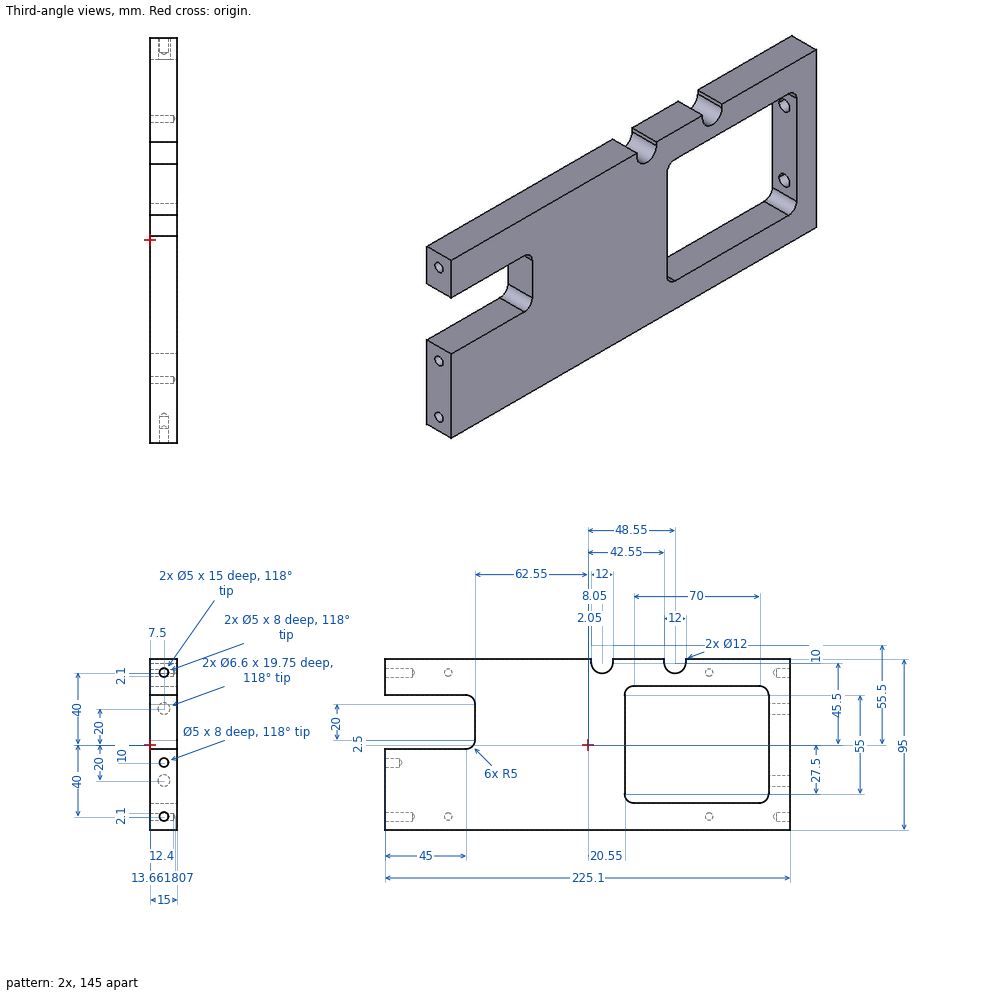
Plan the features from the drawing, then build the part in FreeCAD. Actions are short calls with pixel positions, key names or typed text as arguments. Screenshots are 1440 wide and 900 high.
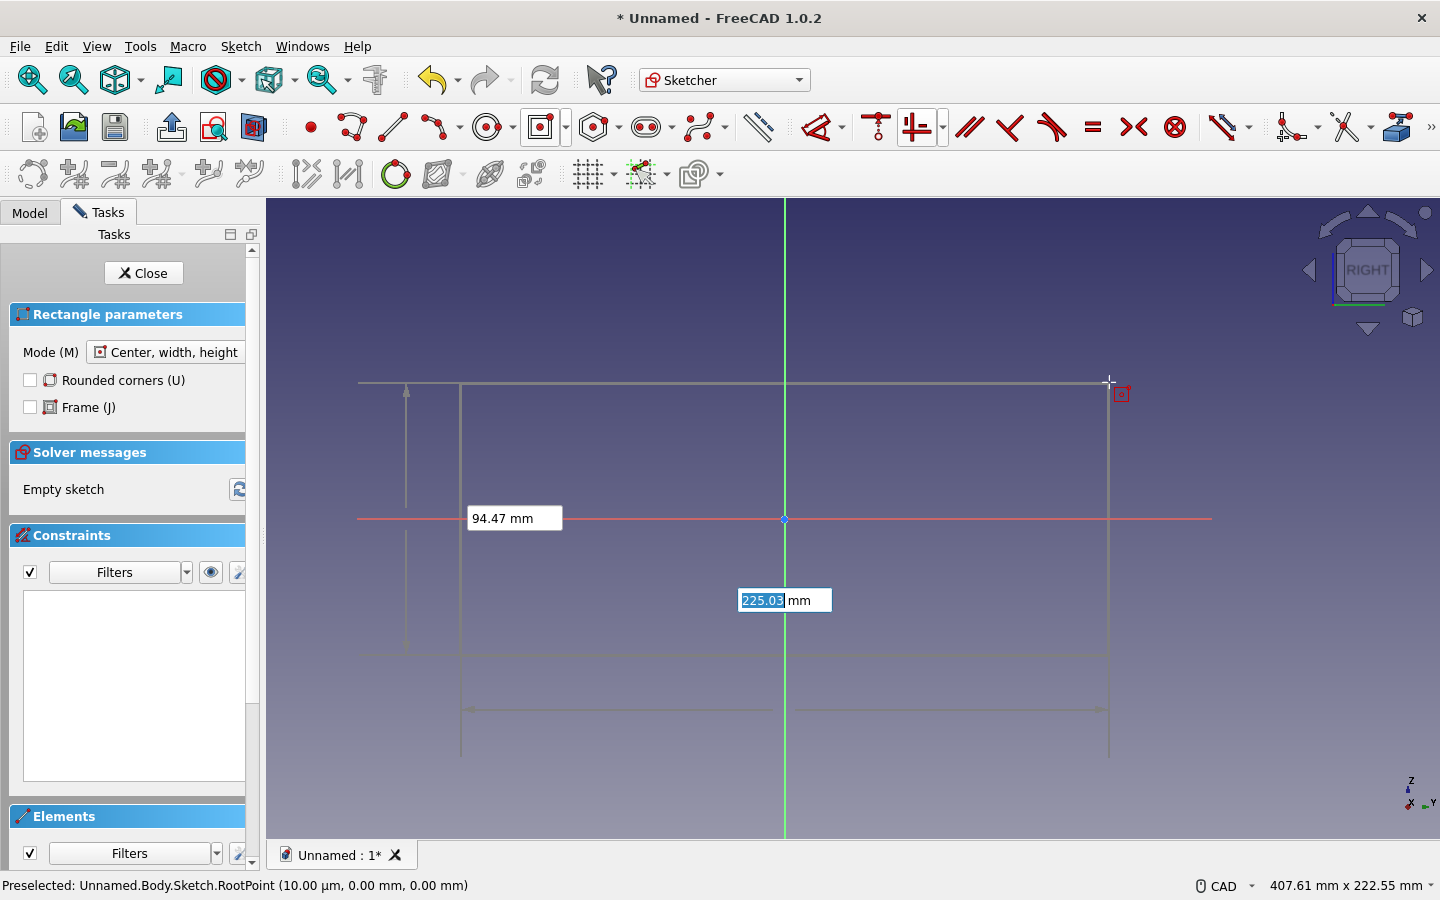
text(225.1)
key(Tab)
text(95)
key(Return)
key(Escape)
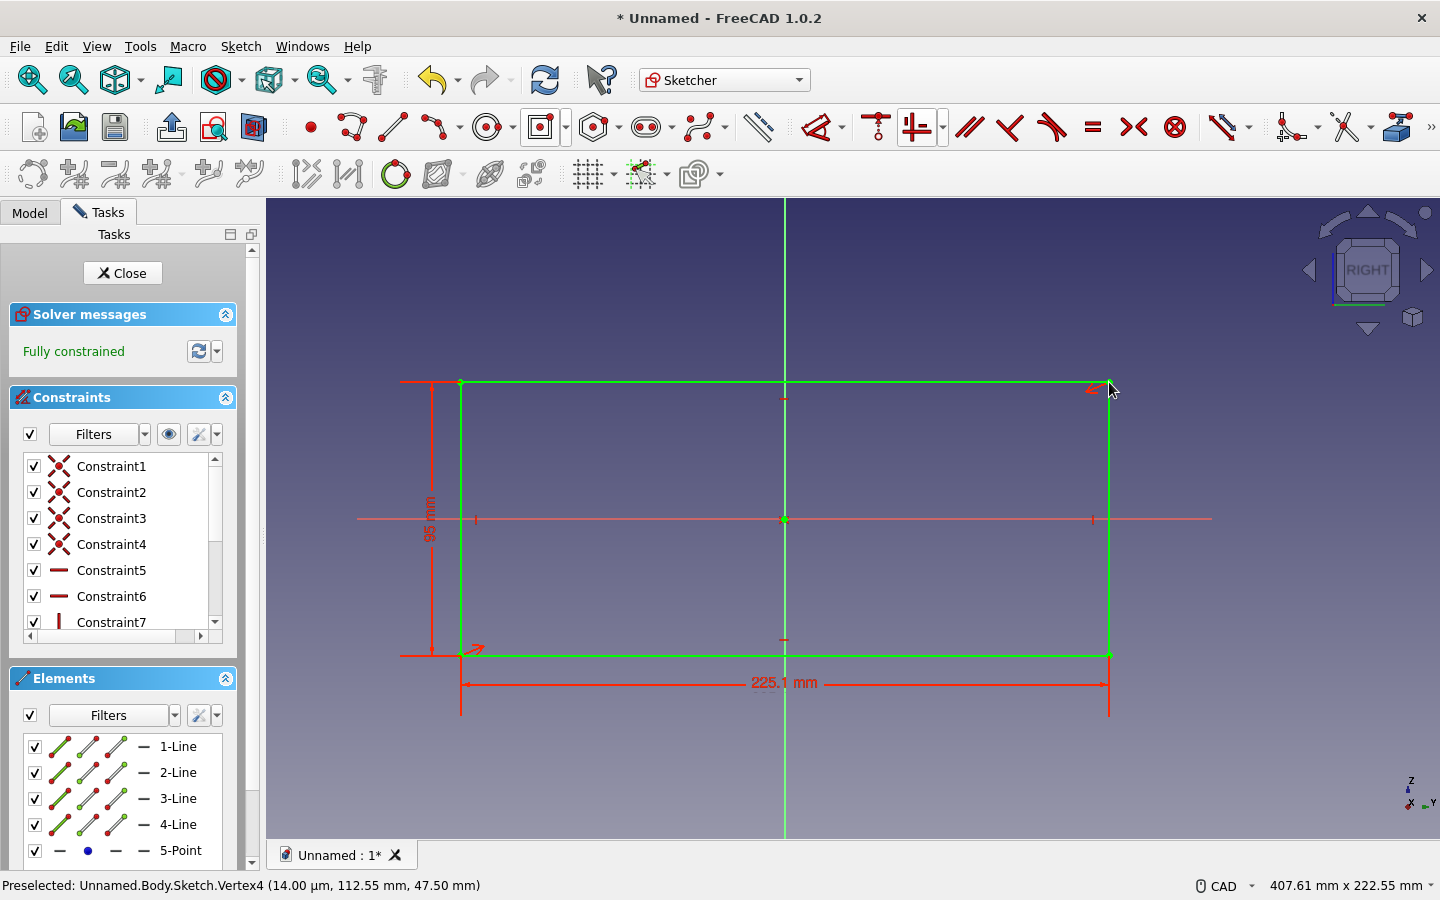
click(123, 273)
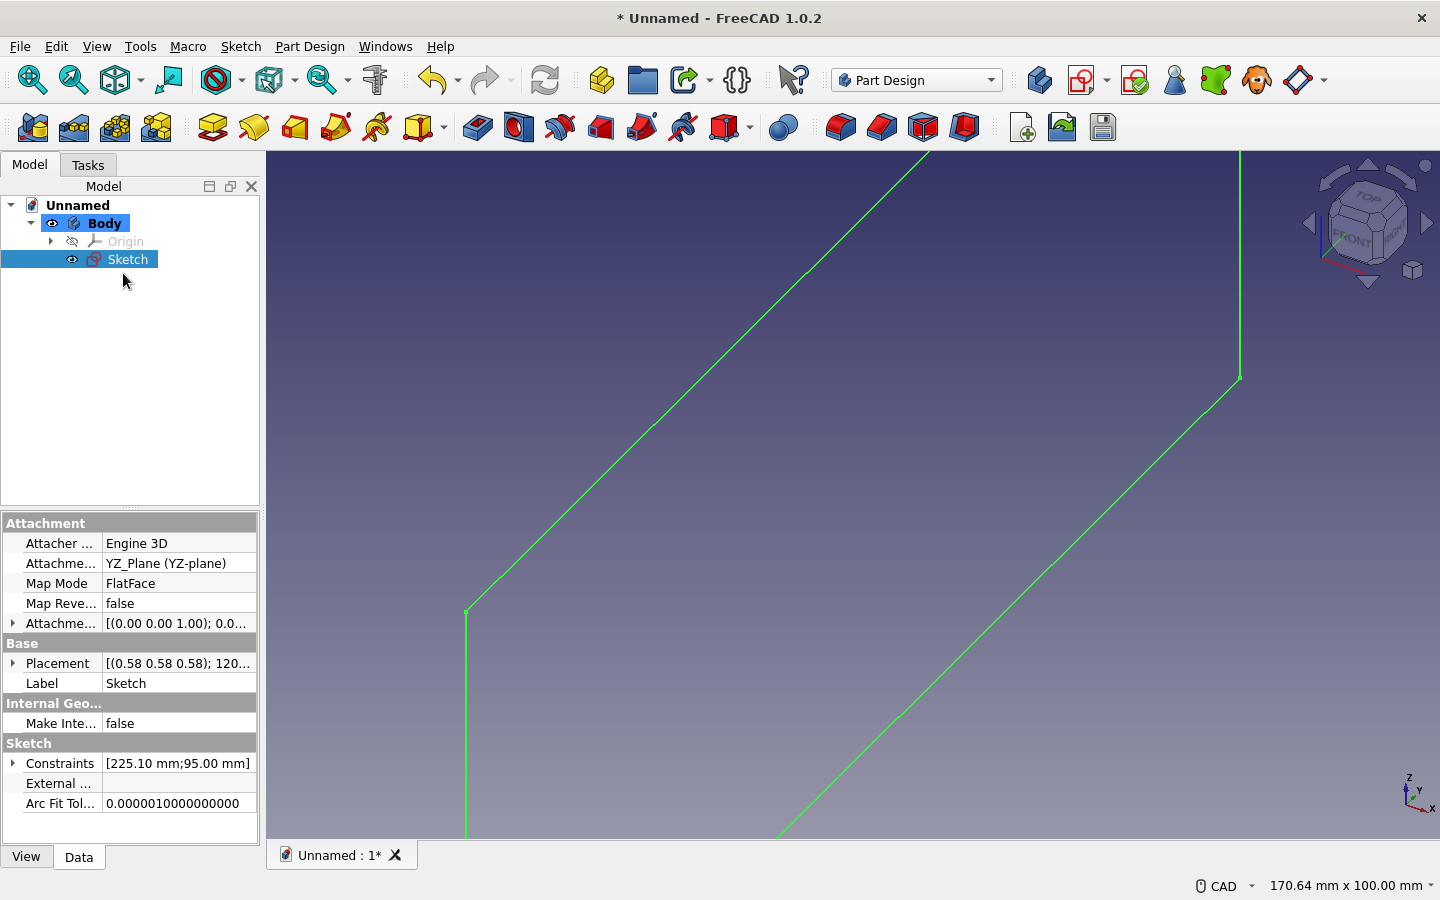
click(213, 128)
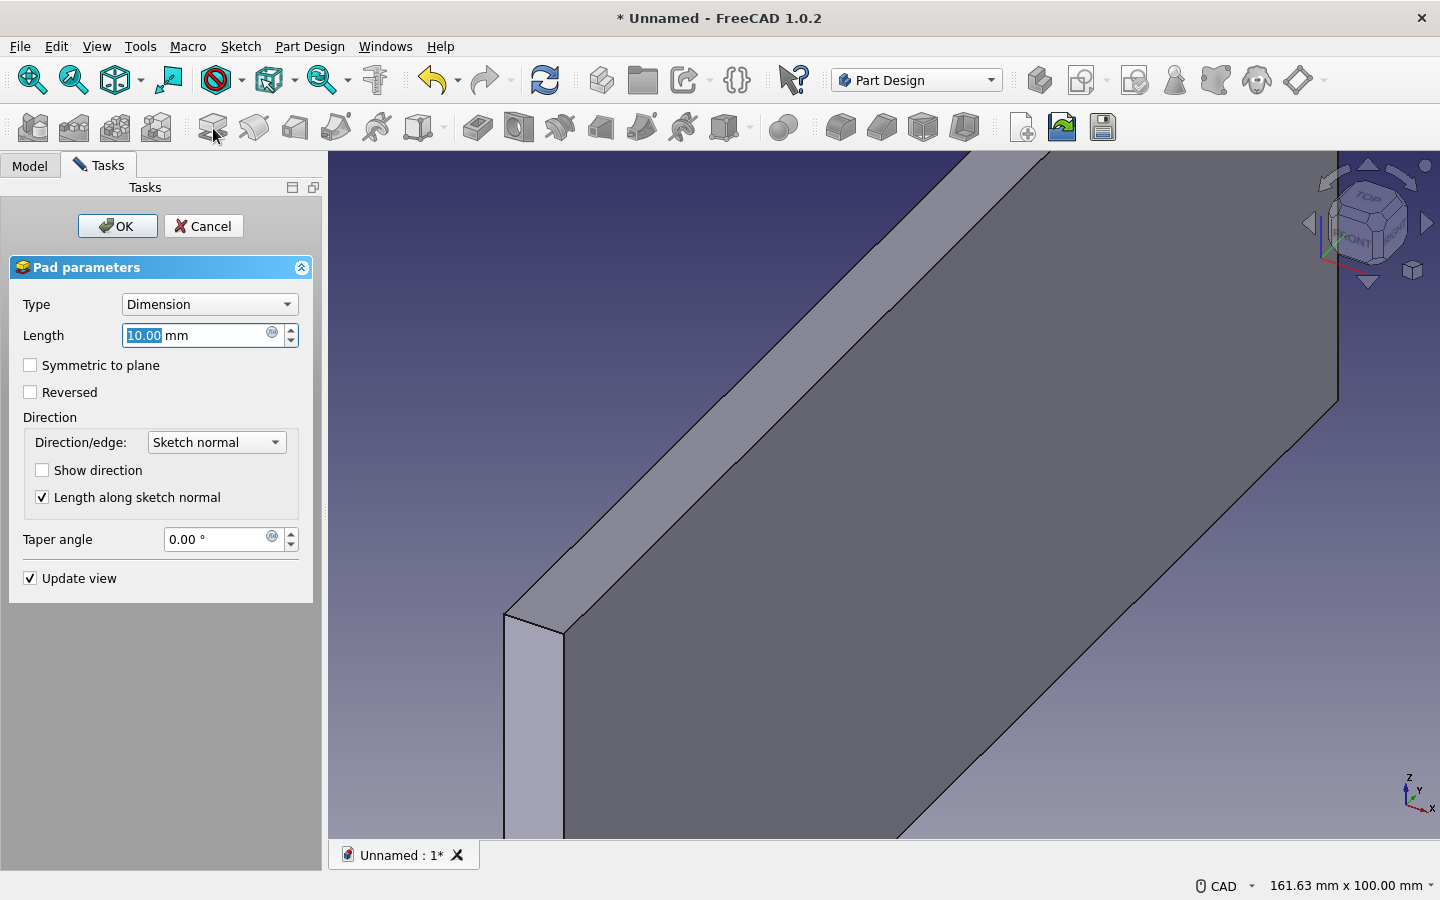
text(15)
key(Tab)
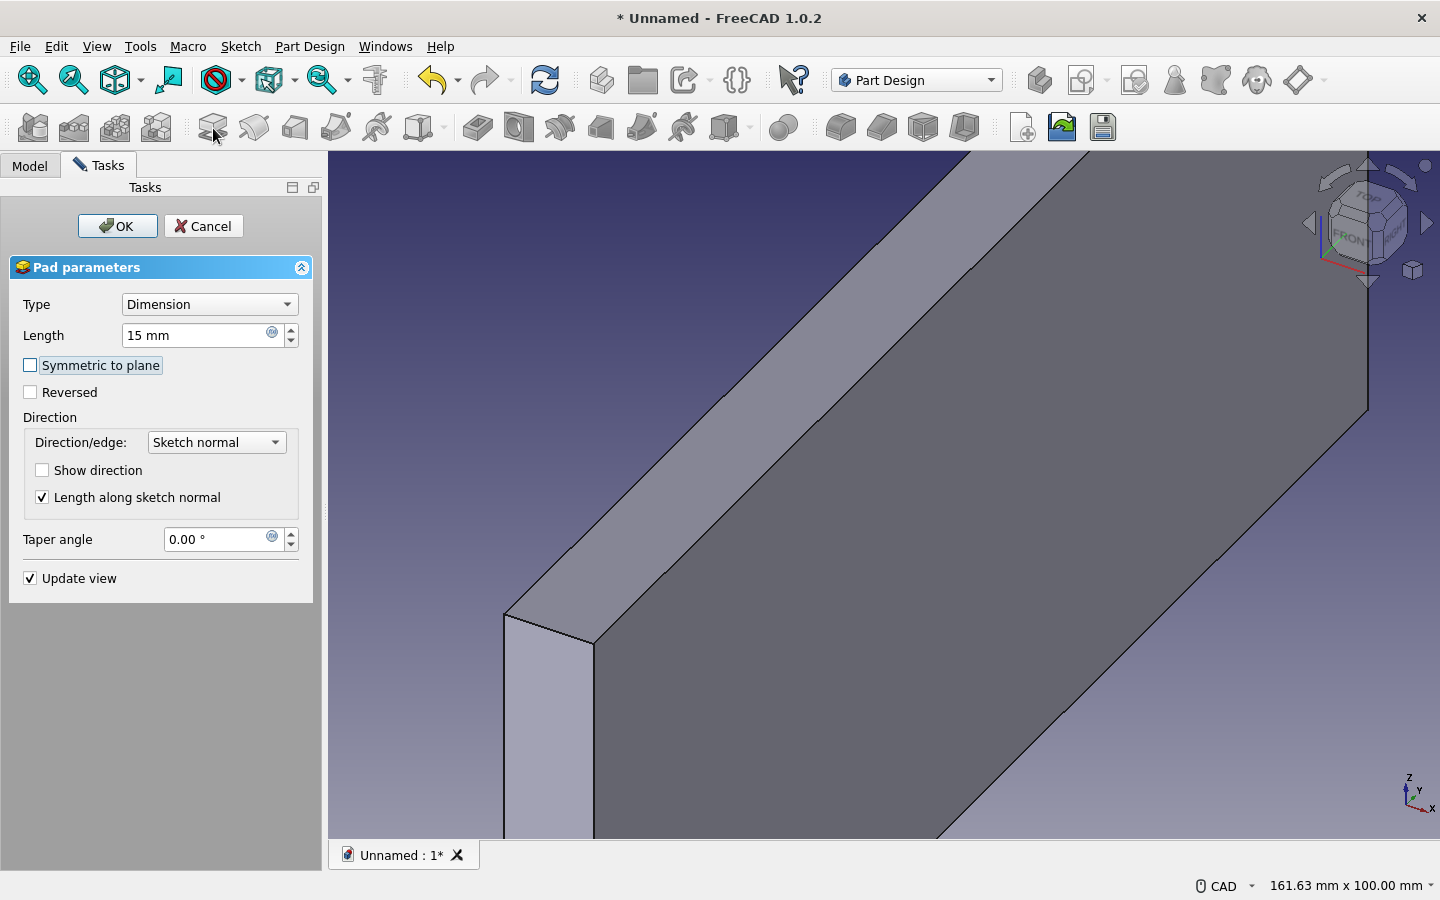
click(118, 226)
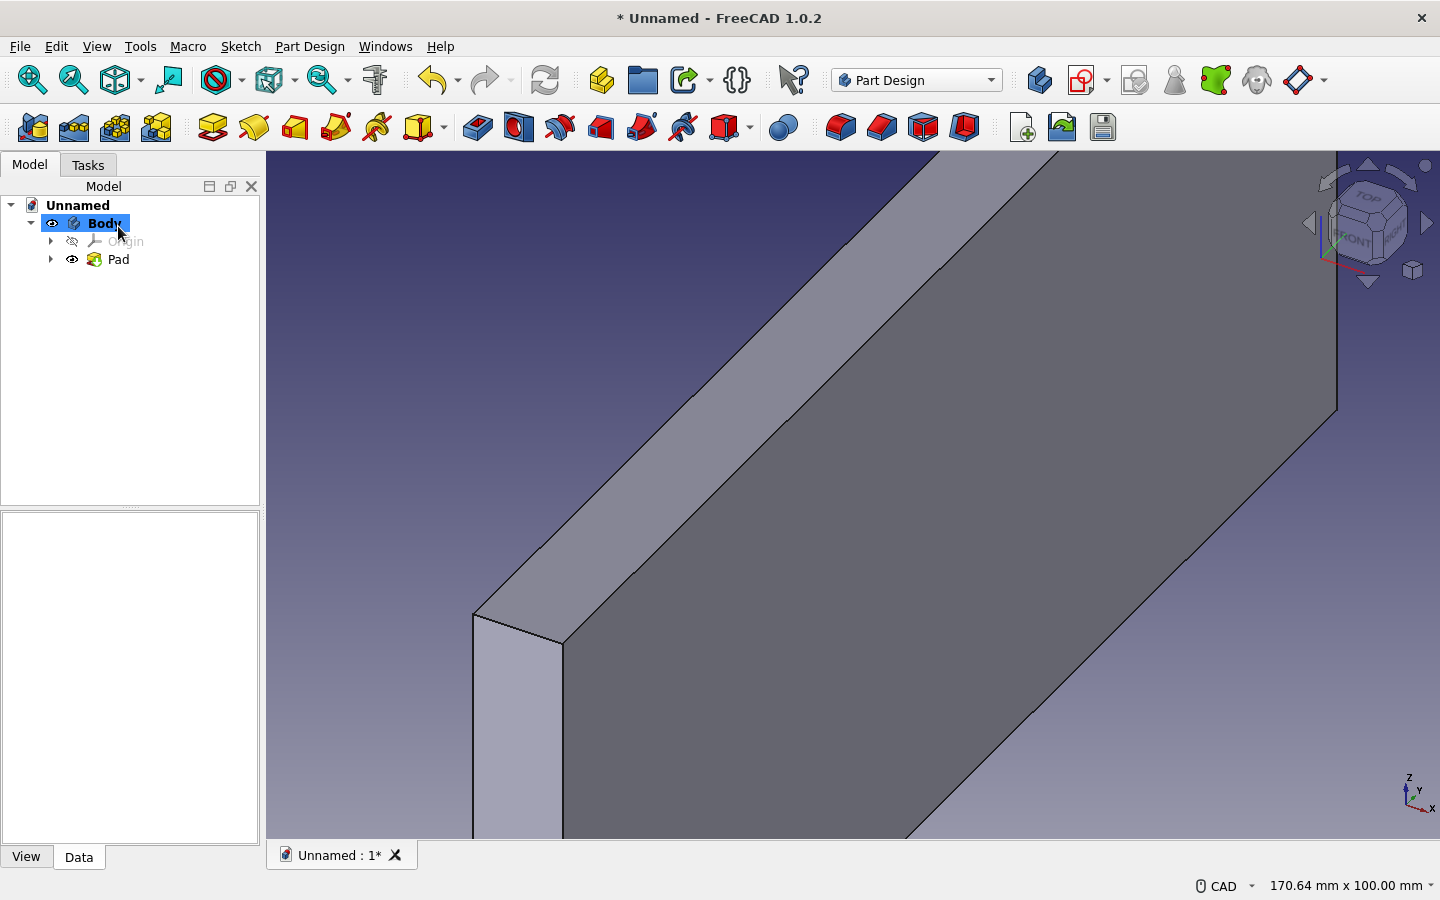
click(33, 80)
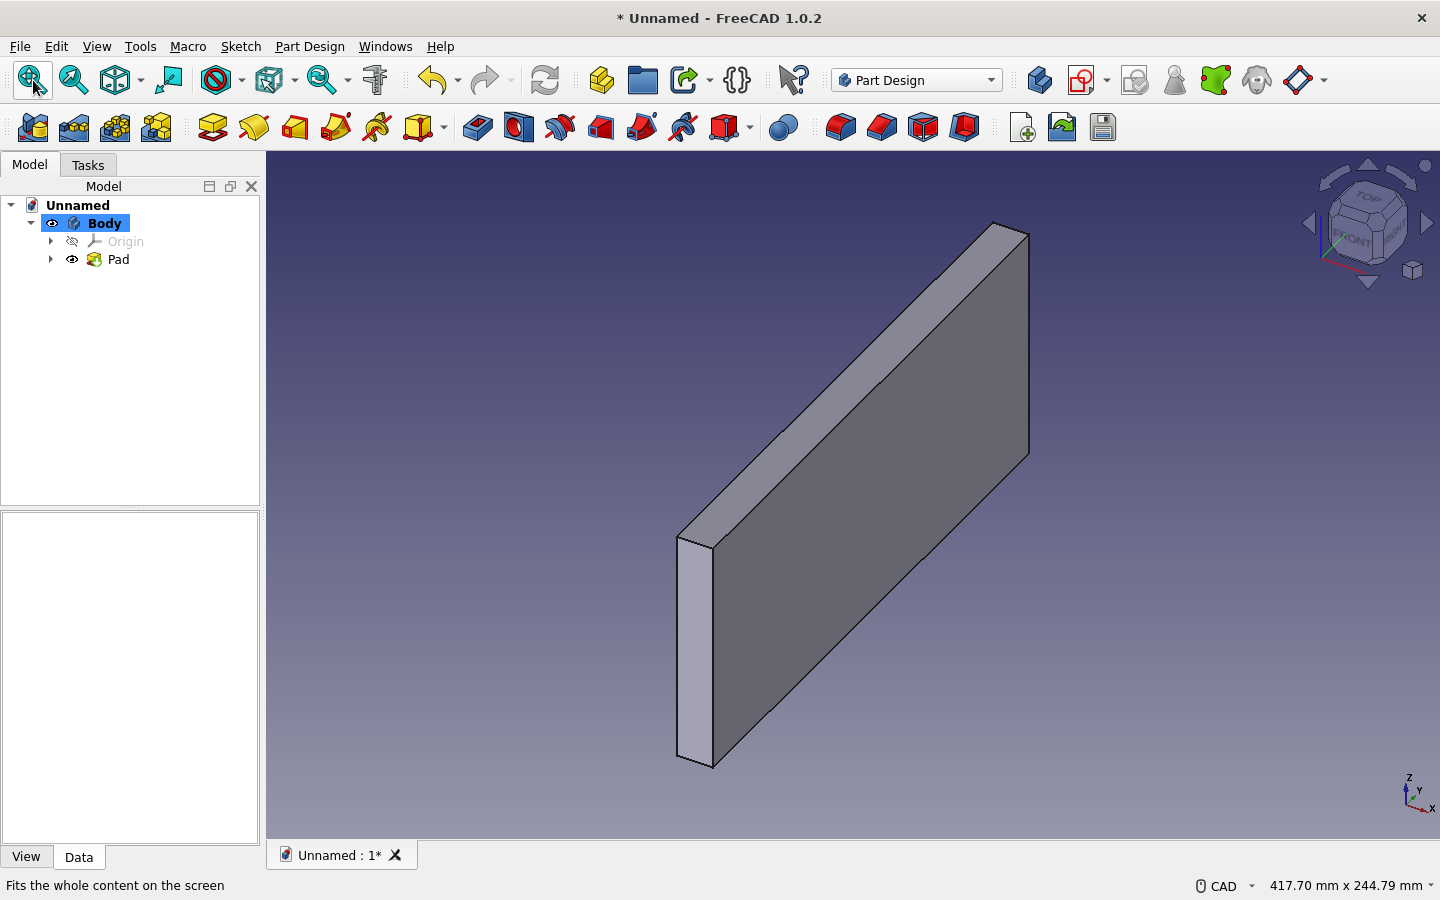
click(1080, 80)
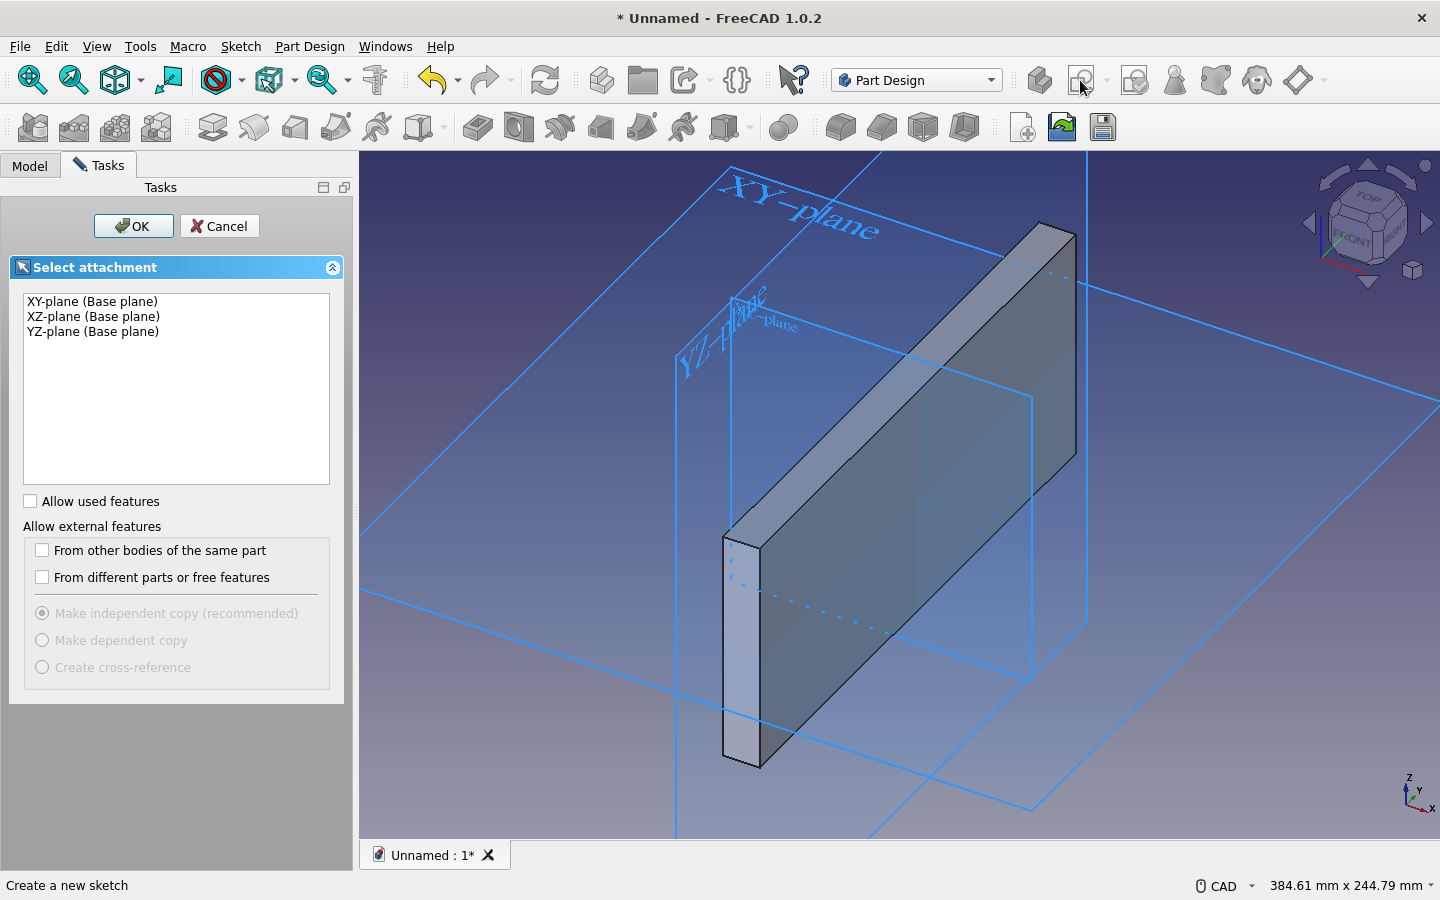
click(84, 332)